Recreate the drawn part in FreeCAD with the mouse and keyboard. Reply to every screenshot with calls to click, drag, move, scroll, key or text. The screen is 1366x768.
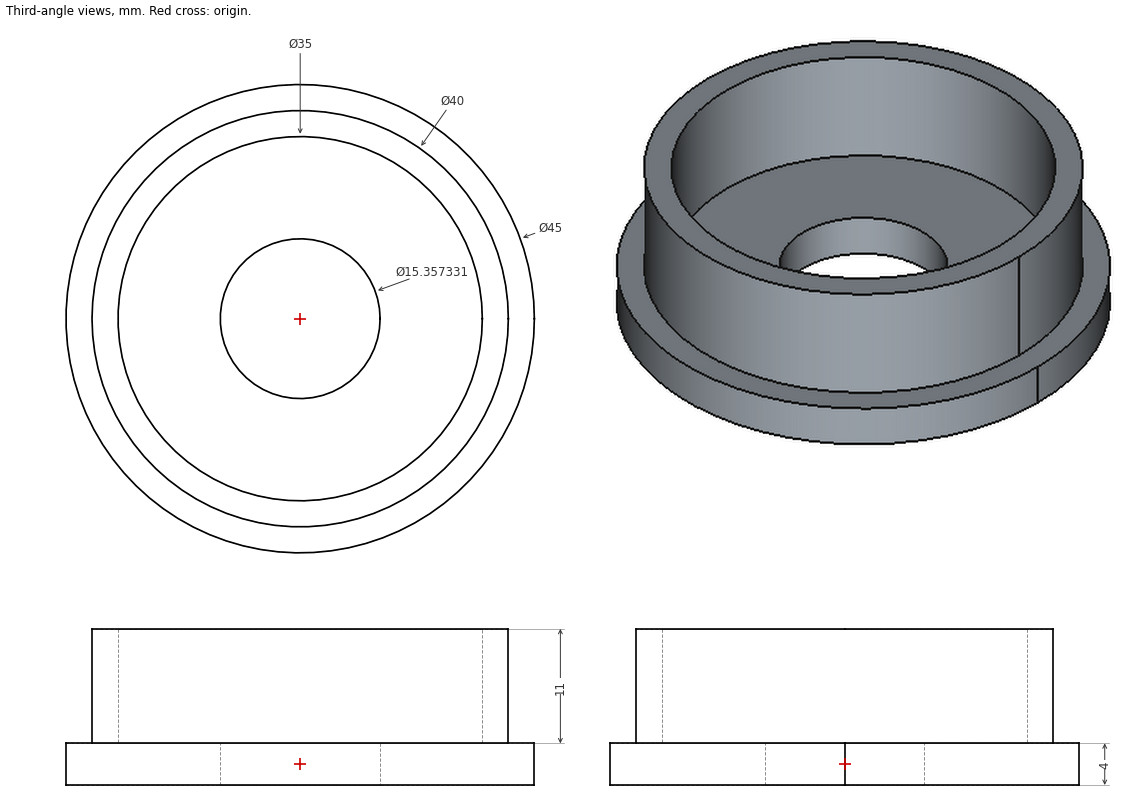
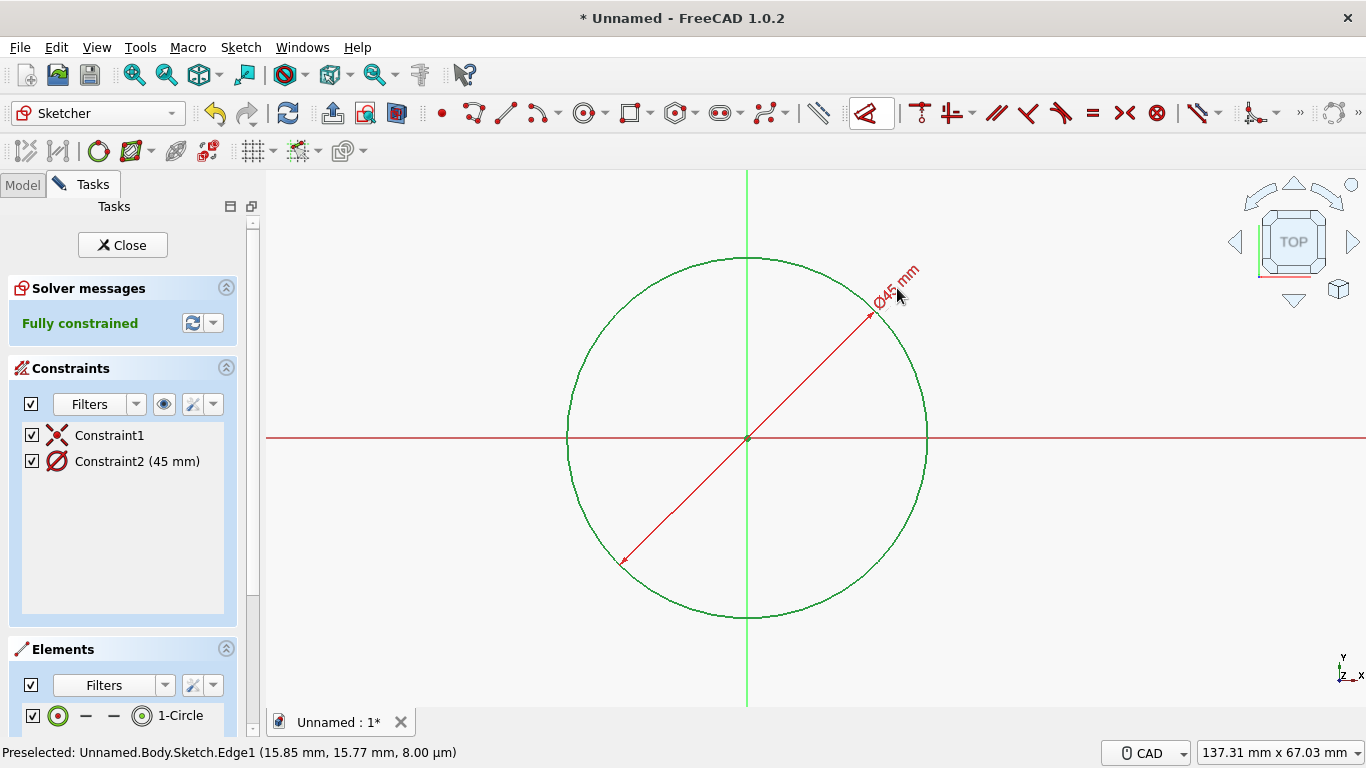
click(123, 245)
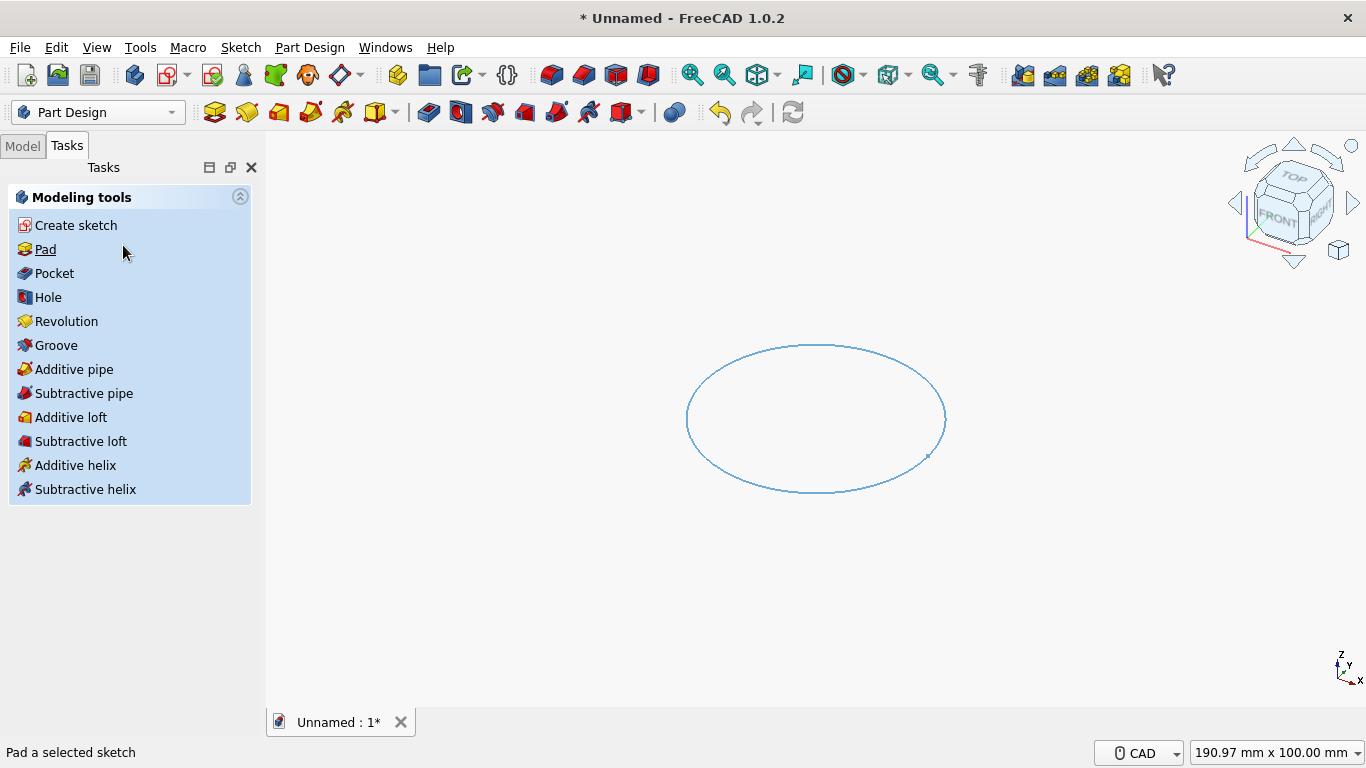
click(216, 112)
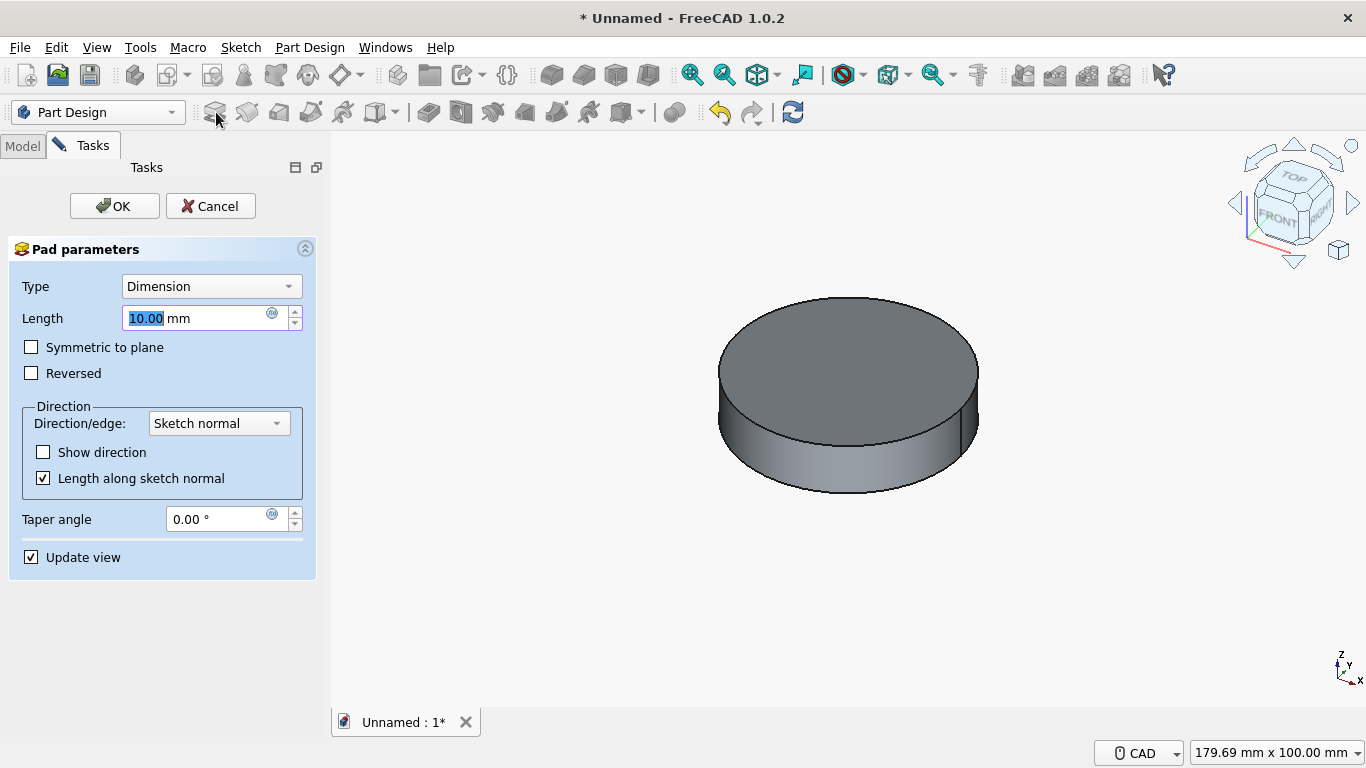
text(4)
key(Tab)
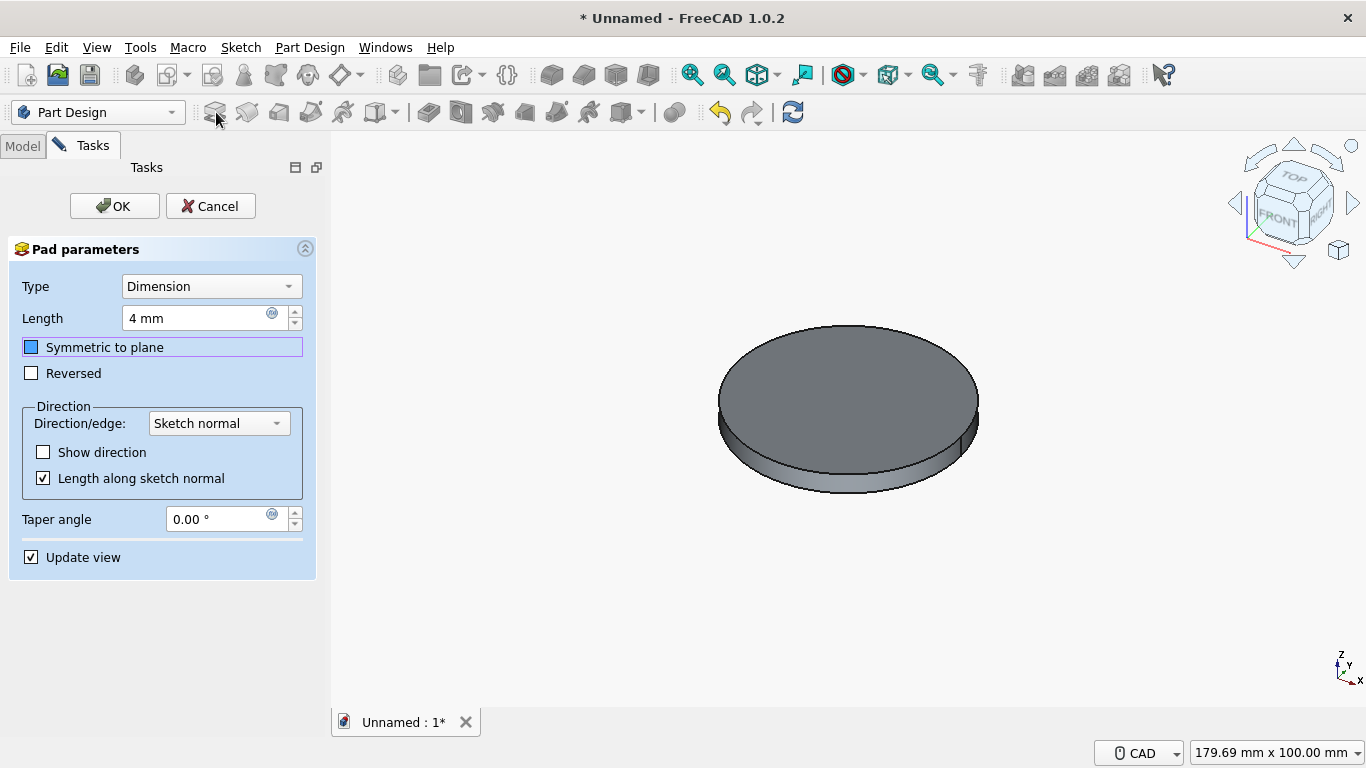
click(30, 347)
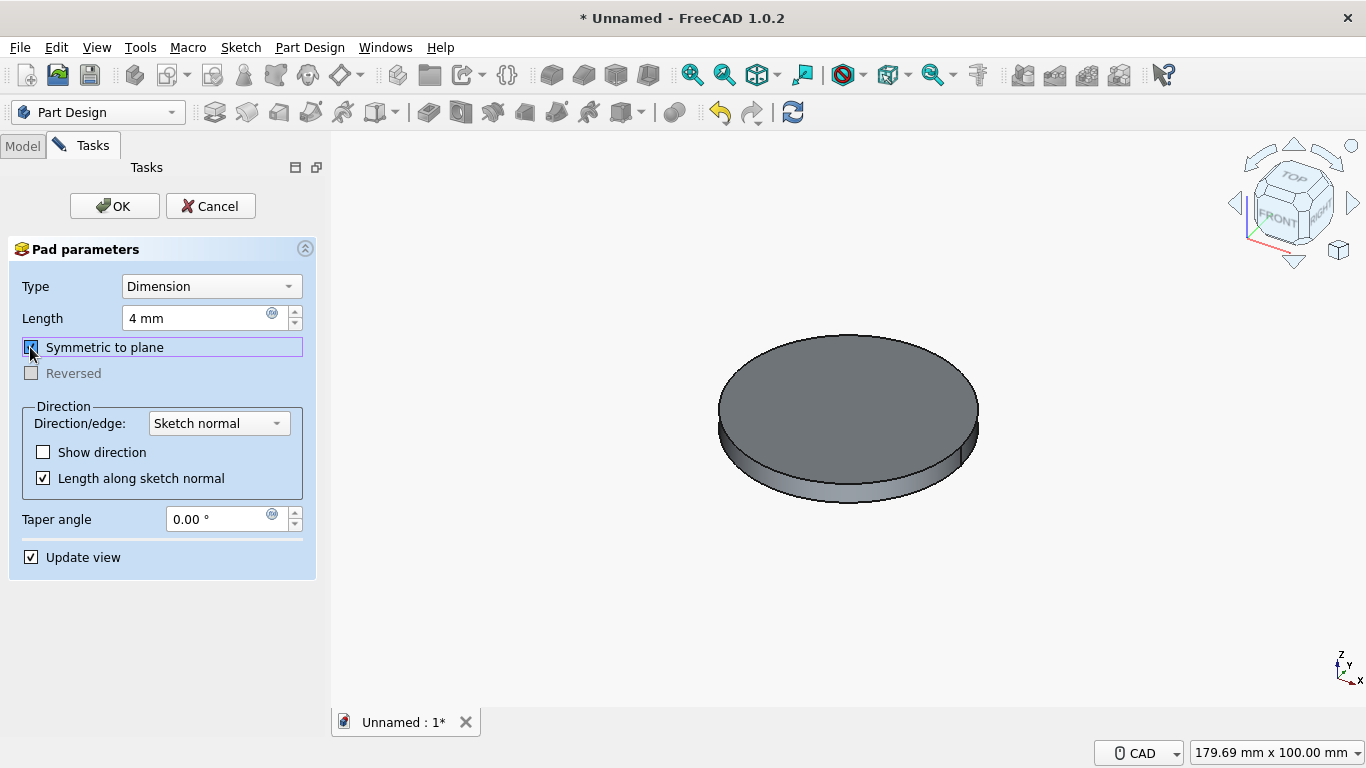
click(115, 206)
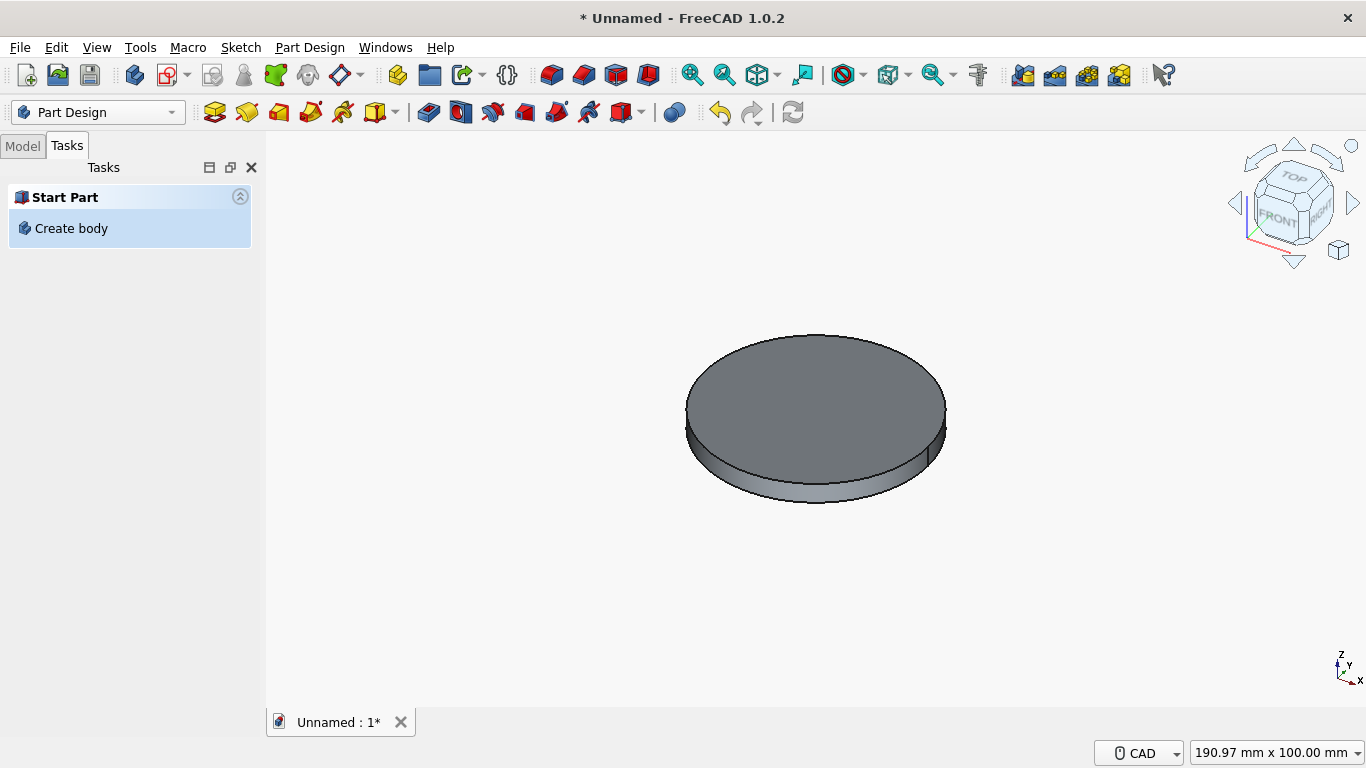
key(v)
key(f)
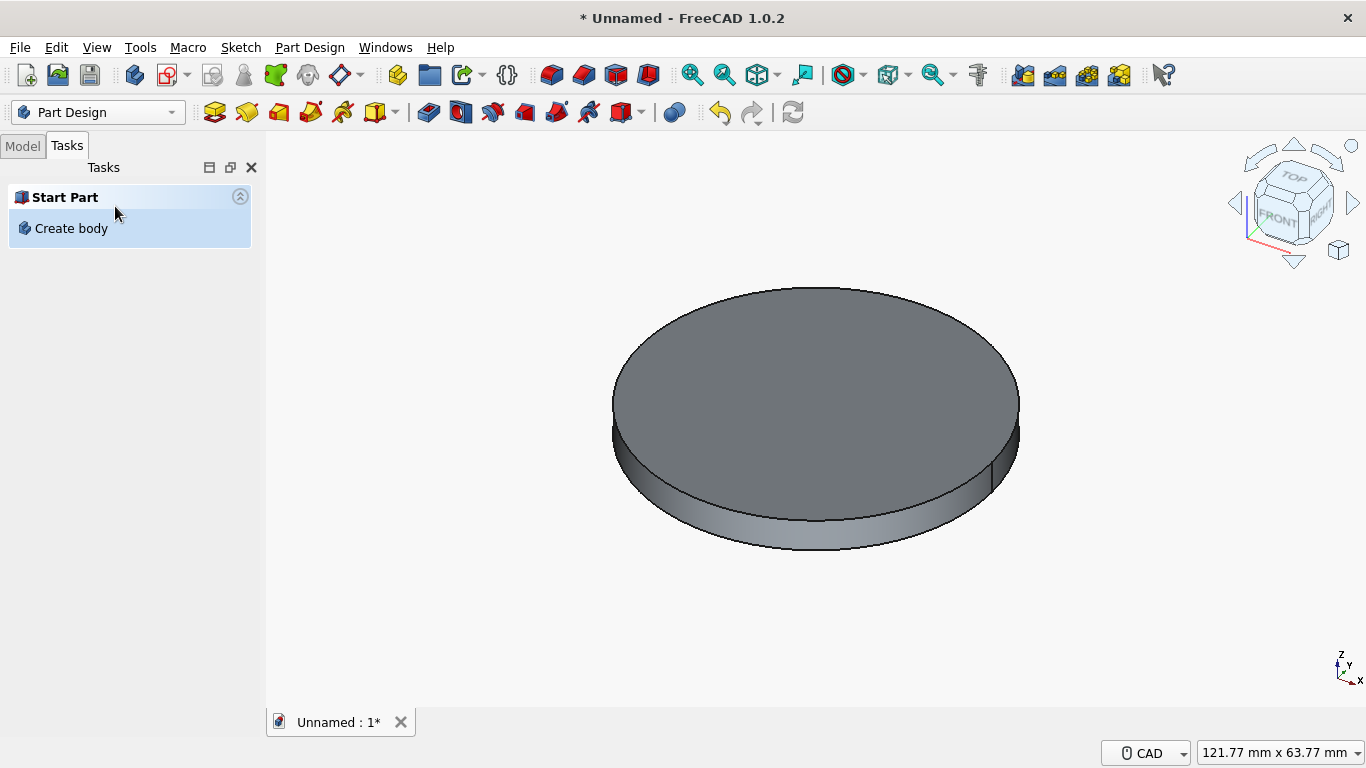
click(816, 403)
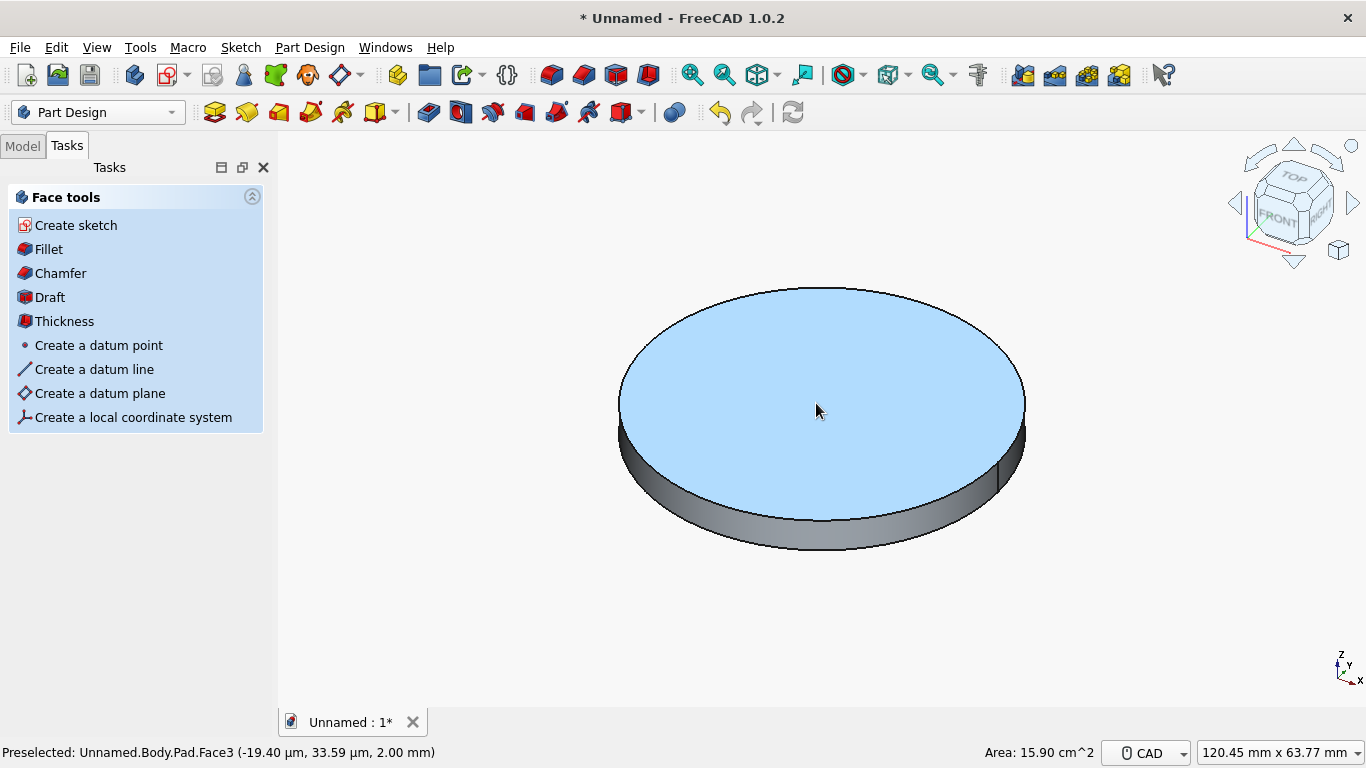
click(168, 76)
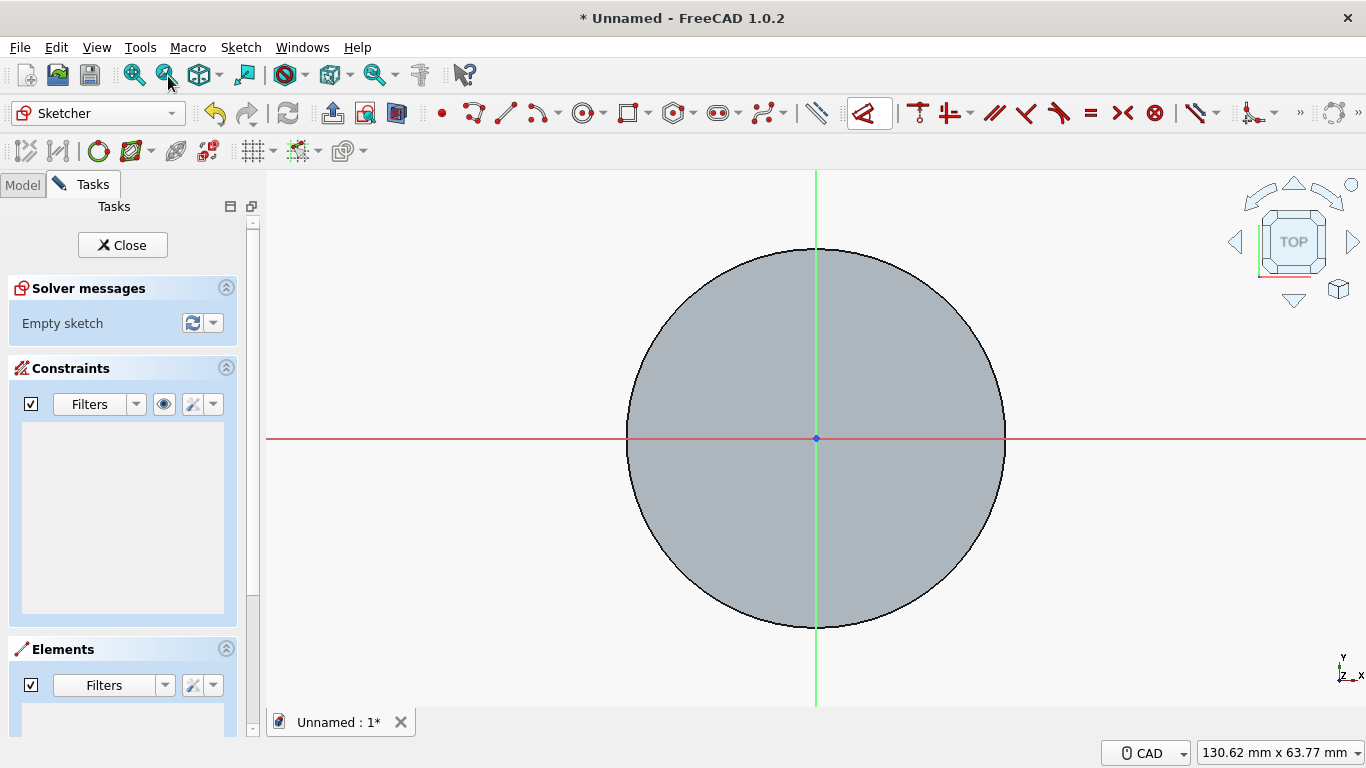
click(584, 114)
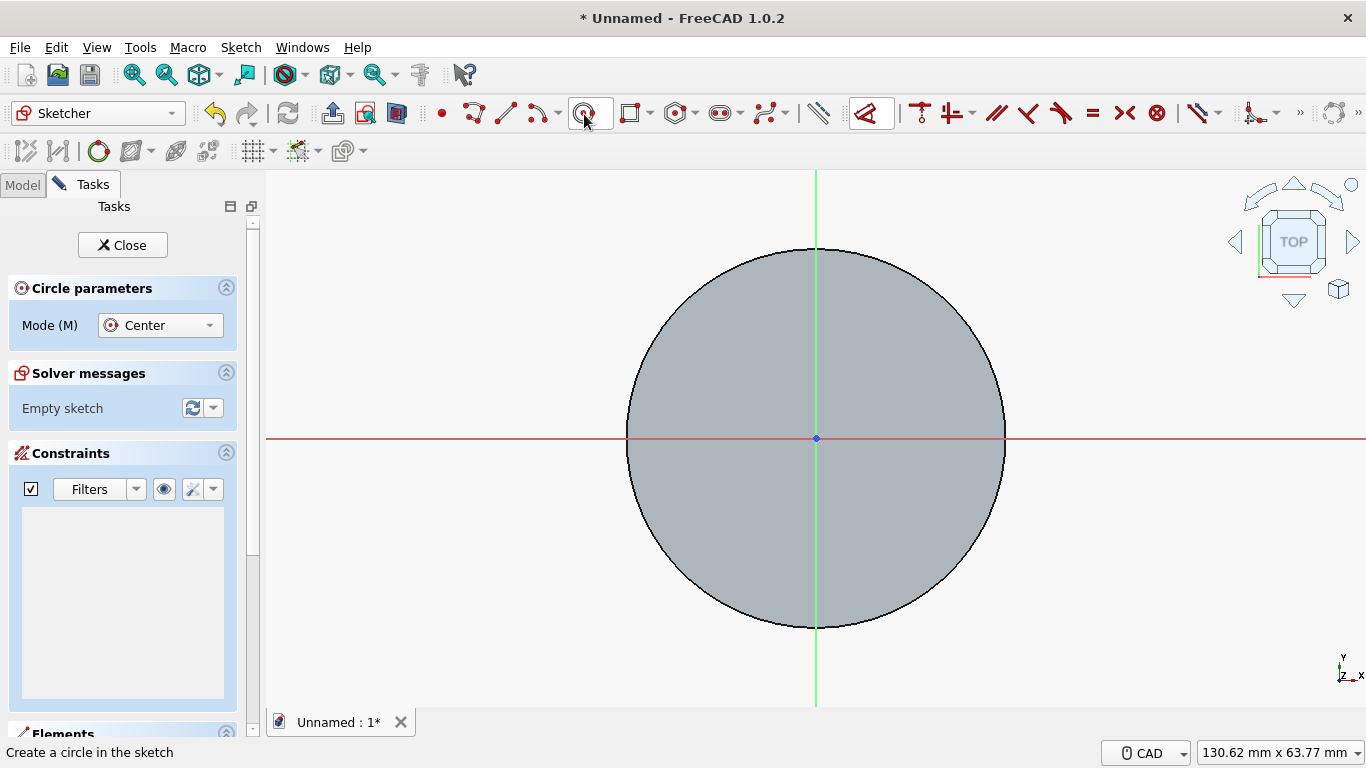
click(816, 438)
click(935, 319)